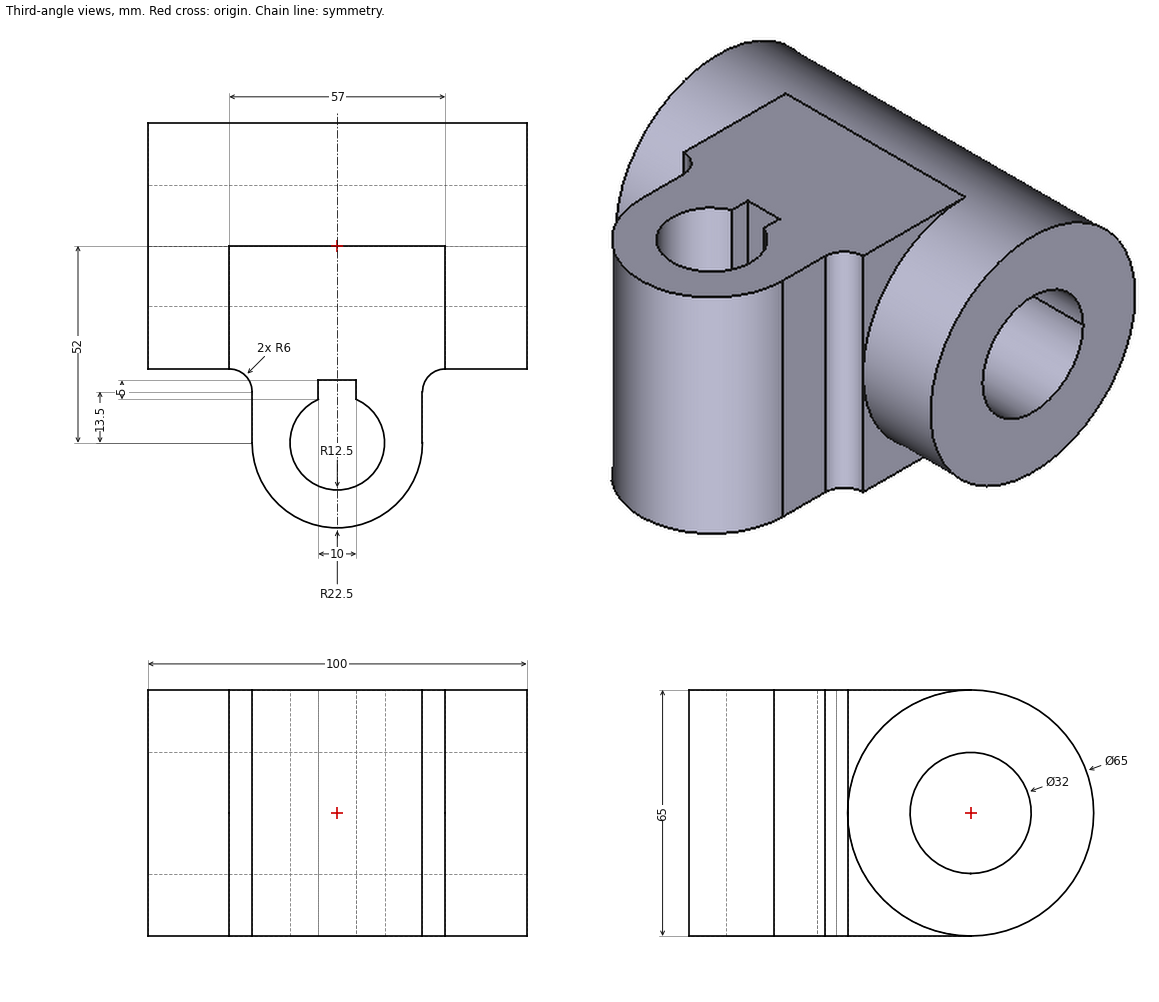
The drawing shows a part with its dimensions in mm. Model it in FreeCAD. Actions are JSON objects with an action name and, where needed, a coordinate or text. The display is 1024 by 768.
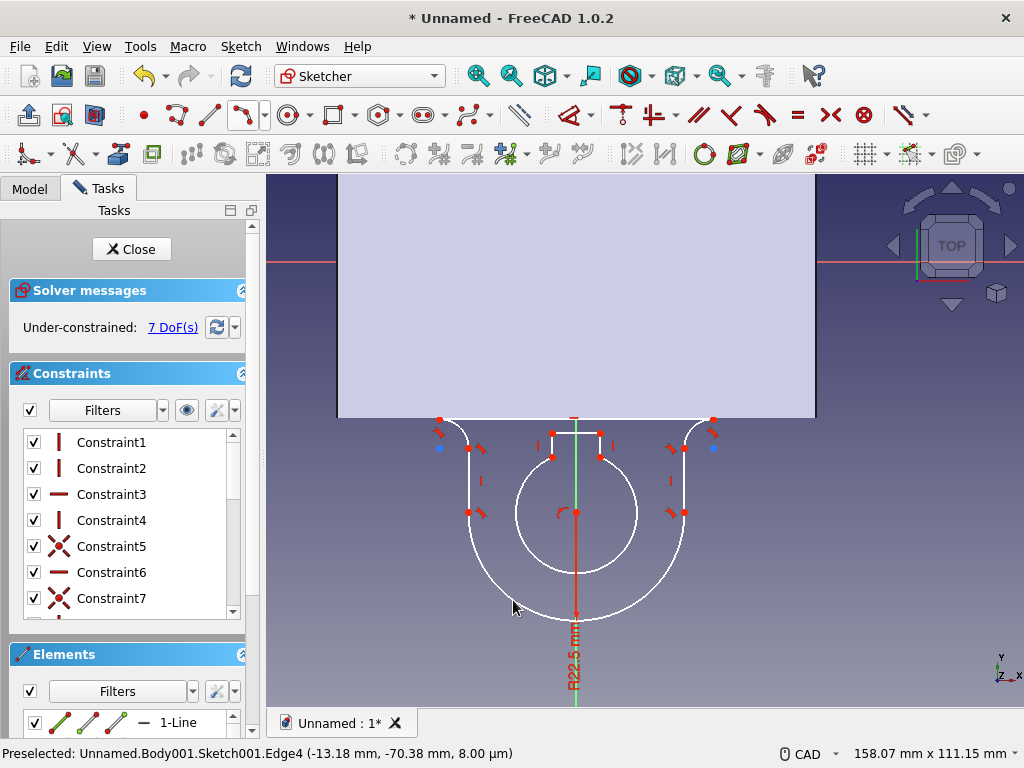
{"action": "scroll", "coordinate": [687, 435], "scroll_direction": "up", "scroll_amount": 2}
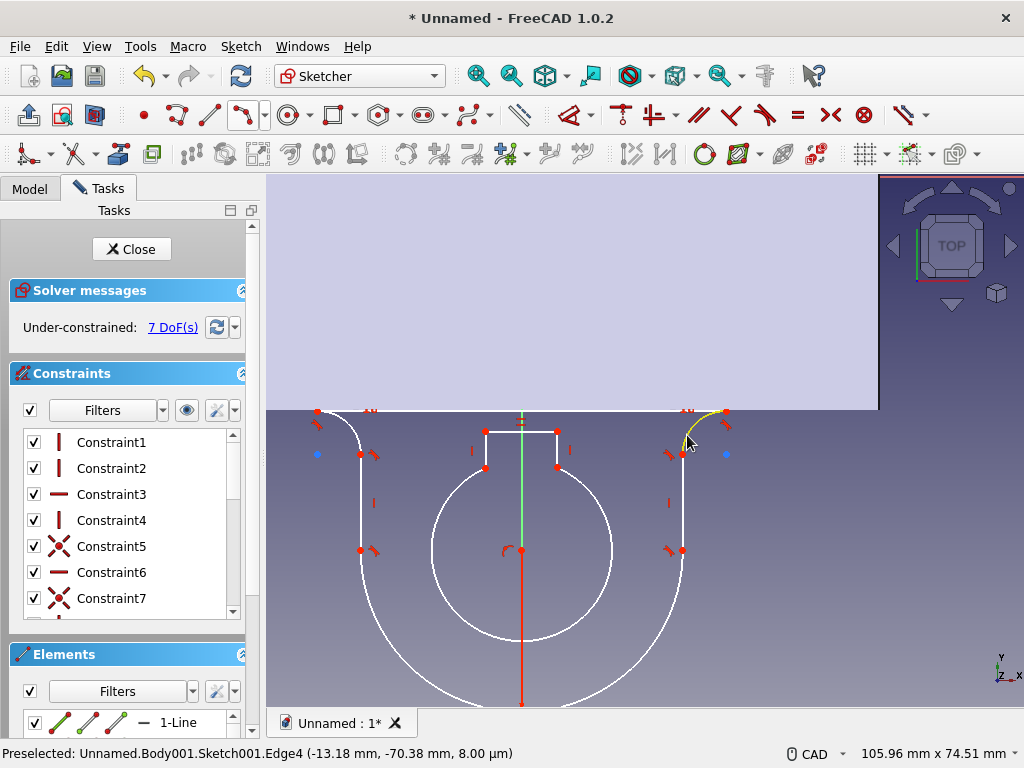
{"action": "left_click", "coordinate": [687, 435]}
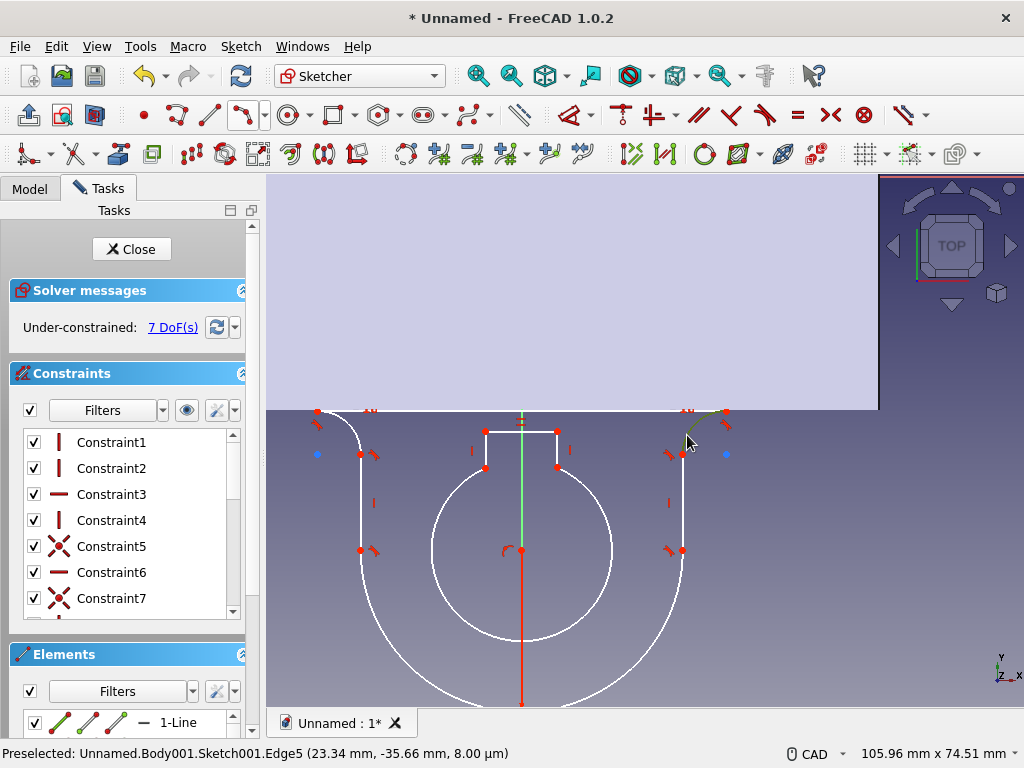
{"action": "left_click", "coordinate": [590, 116]}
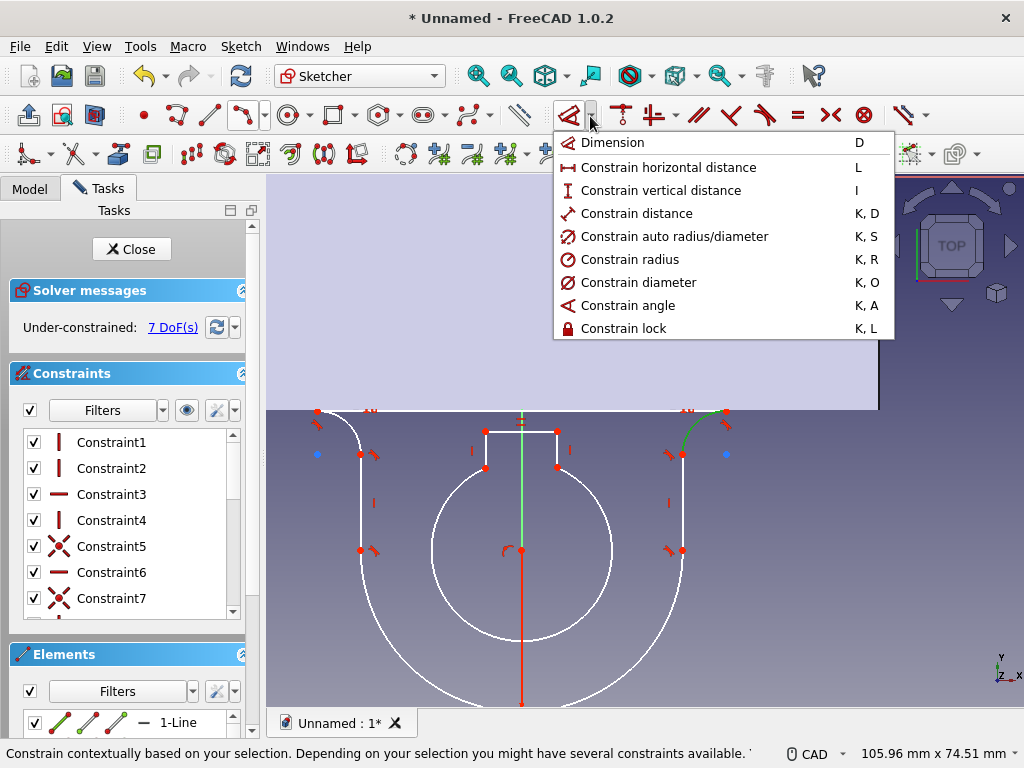
{"action": "left_click", "coordinate": [724, 260]}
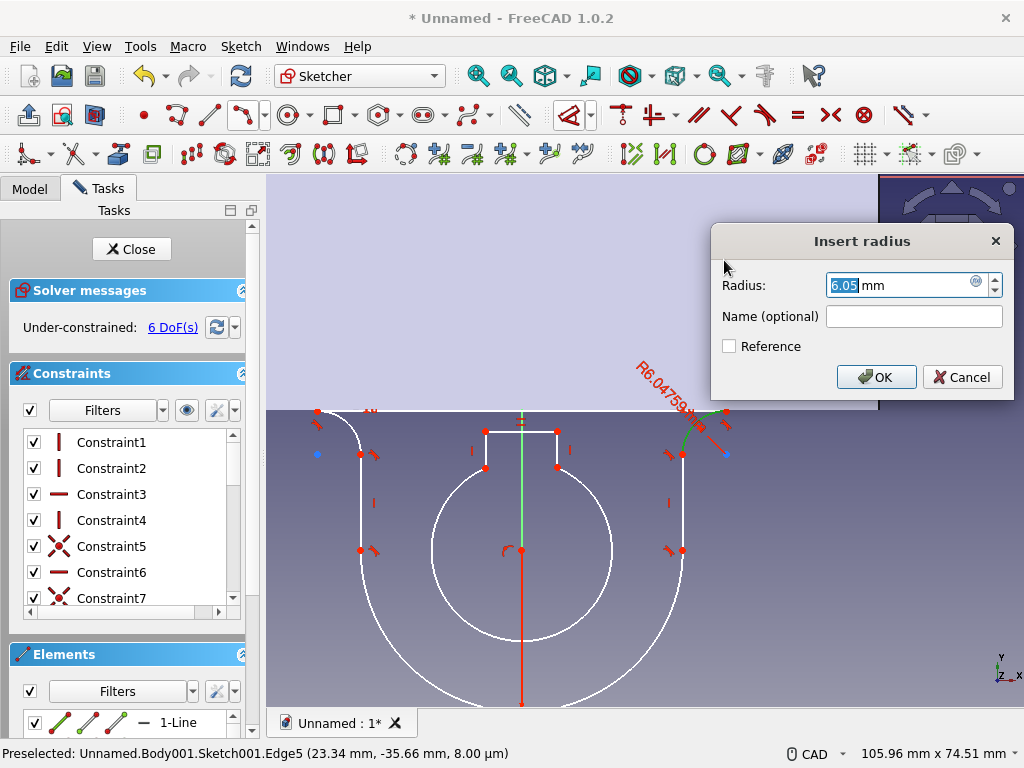
{"action": "type", "text": "6"}
{"action": "key", "text": "Return"}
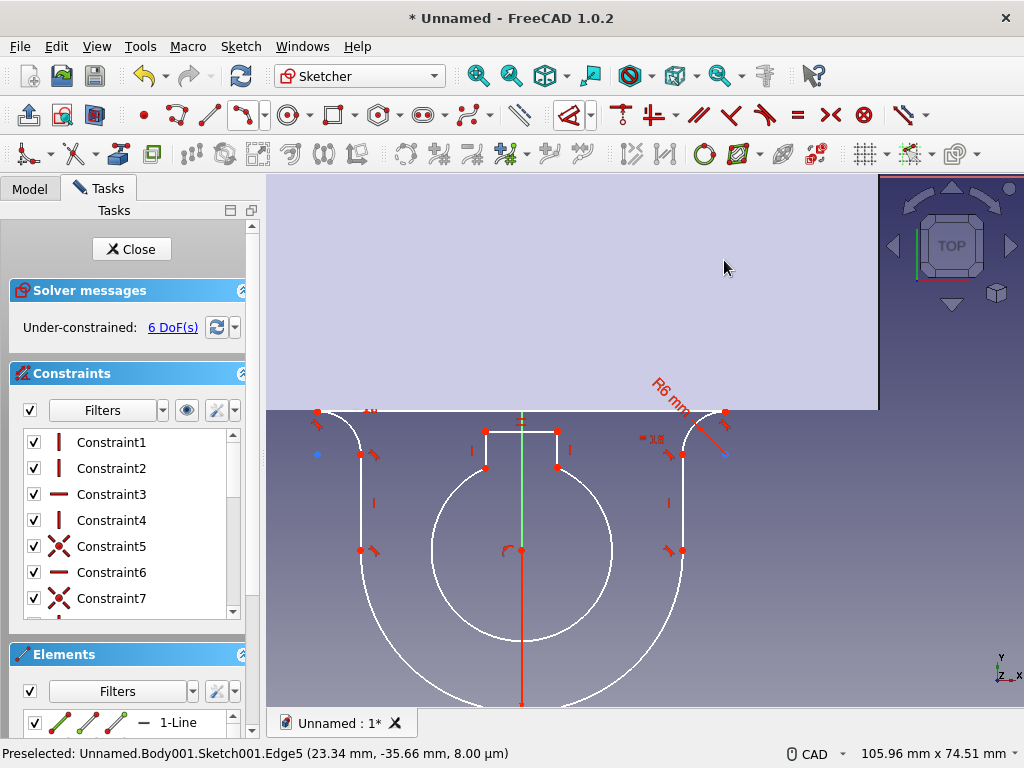
{"action": "left_click", "coordinate": [442, 593]}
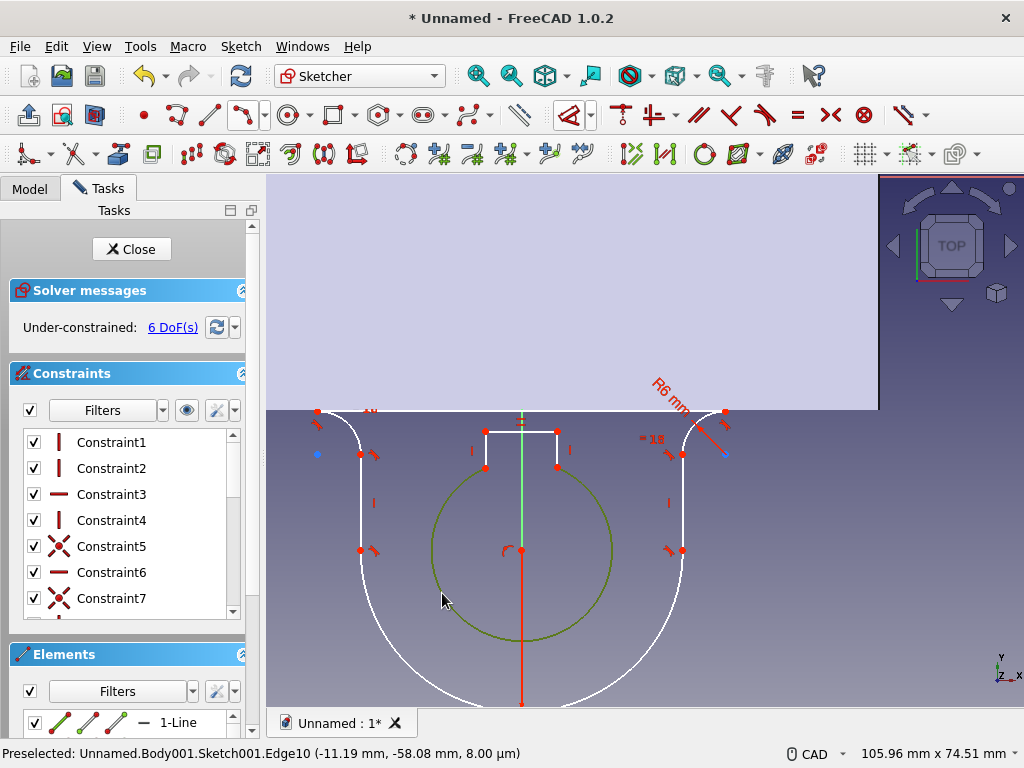
{"action": "key", "text": "k r"}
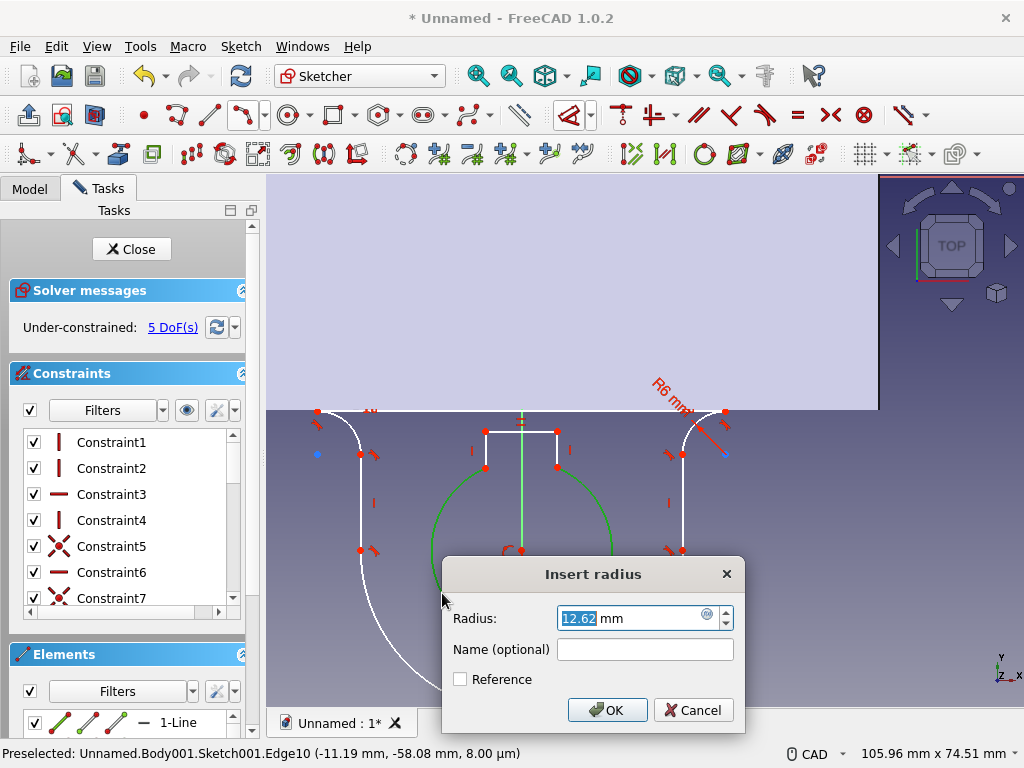
{"action": "type", "text": "12.5"}
{"action": "key", "text": "Return"}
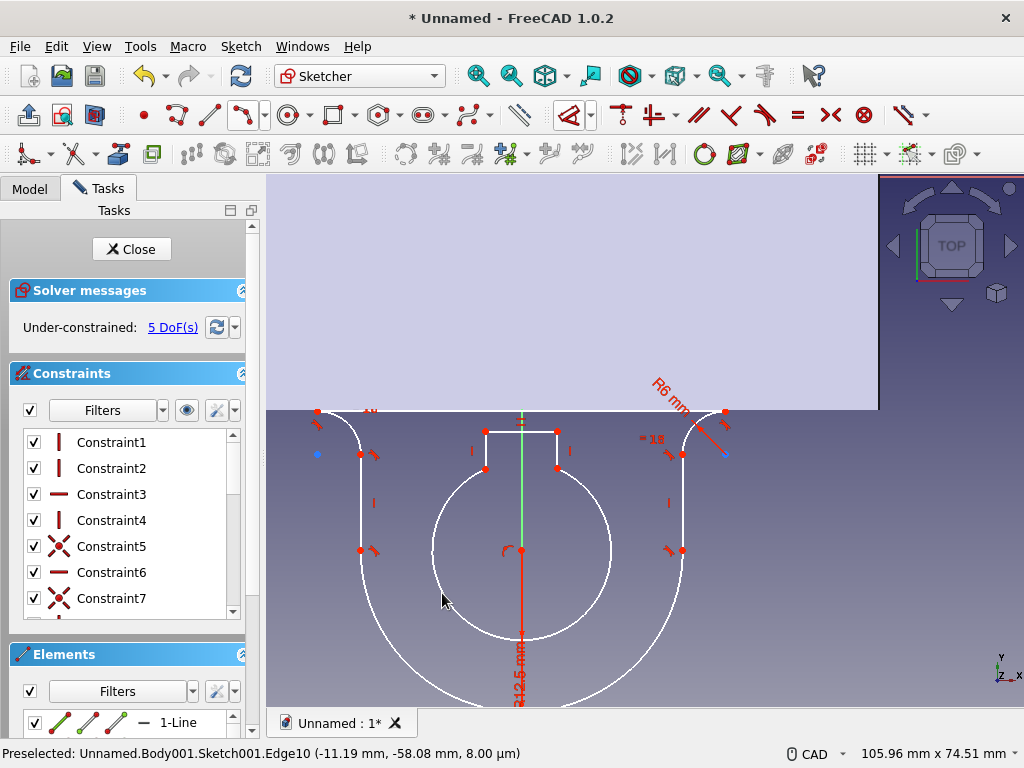
{"action": "scroll", "coordinate": [486, 458], "scroll_direction": "up", "scroll_amount": 2}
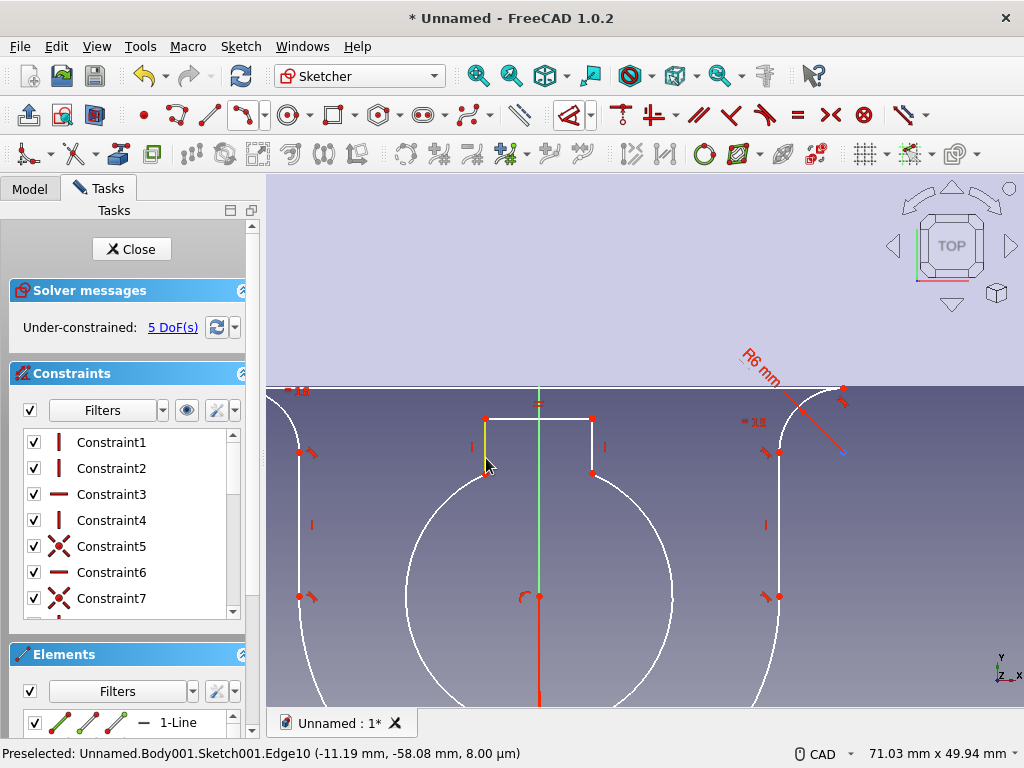
{"action": "left_click", "coordinate": [485, 458]}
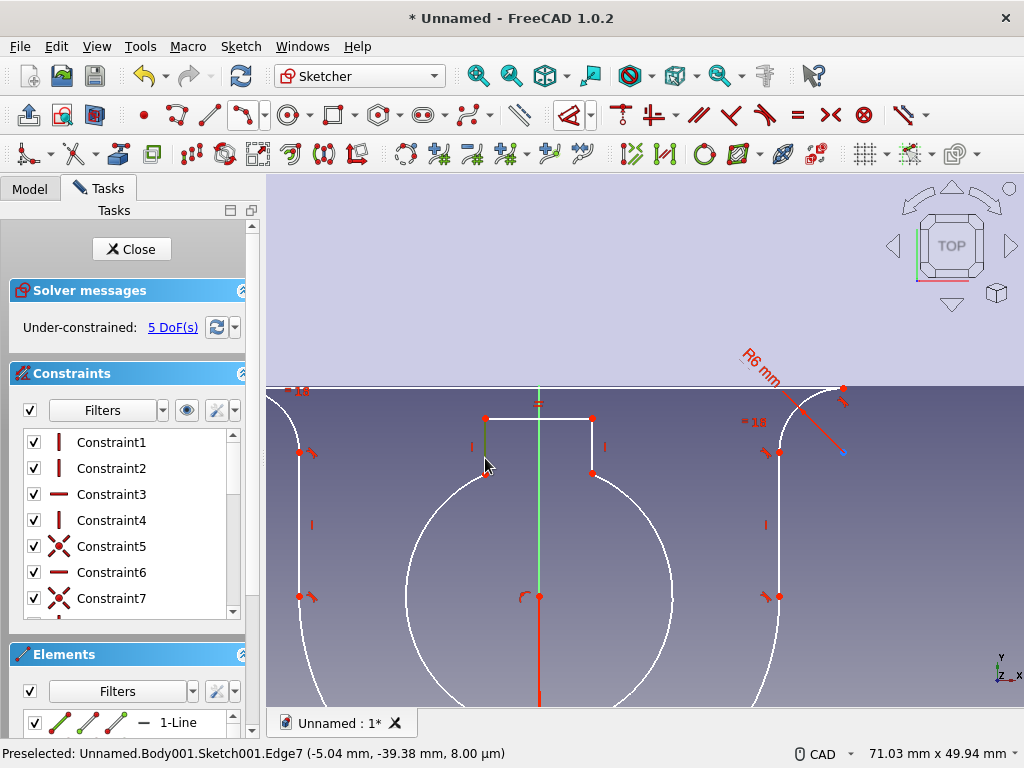
{"action": "key", "text": "i"}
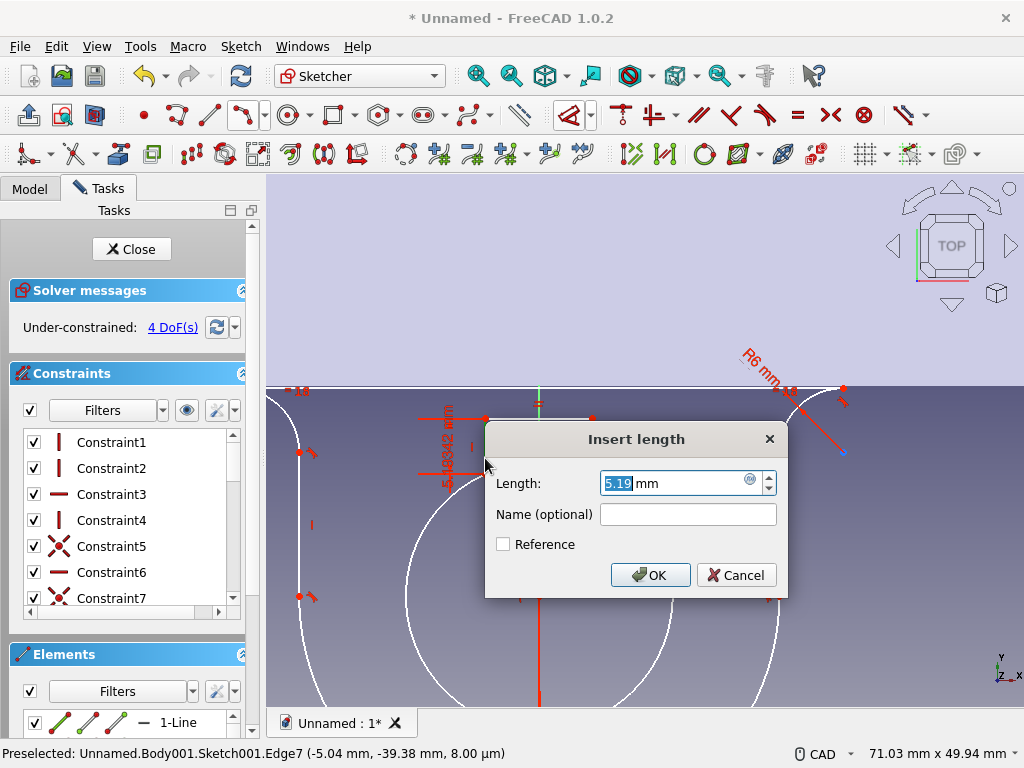
{"action": "type", "text": "5"}
{"action": "key", "text": "Return"}